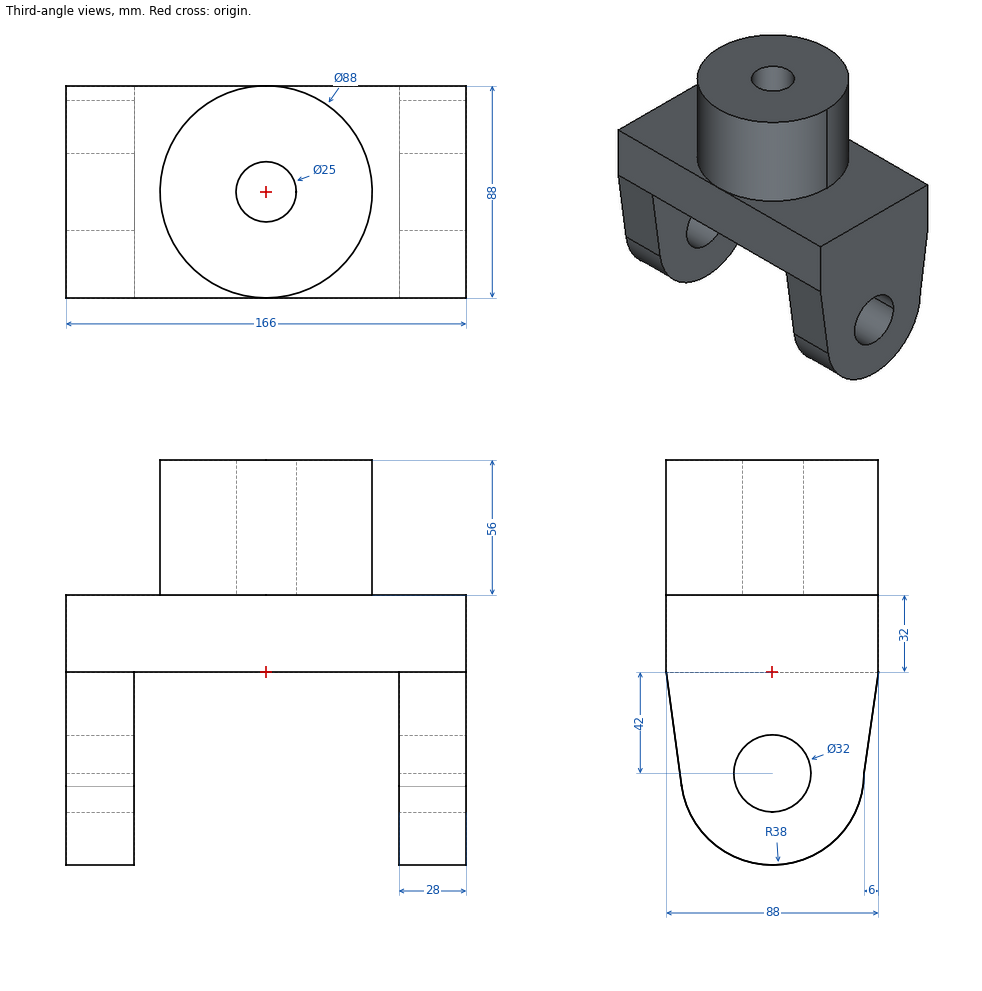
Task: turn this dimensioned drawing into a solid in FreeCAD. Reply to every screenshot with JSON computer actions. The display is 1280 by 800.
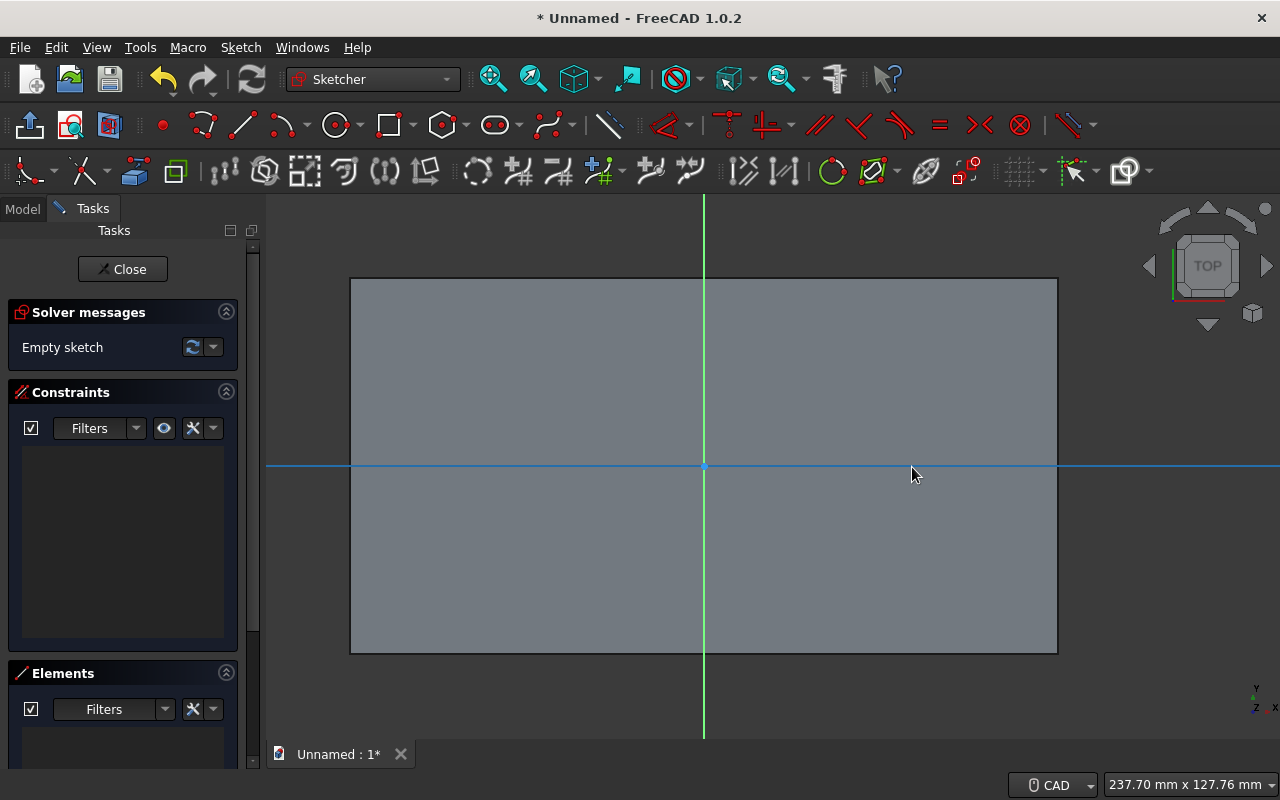
{"action": "left_click", "coordinate": [336, 126]}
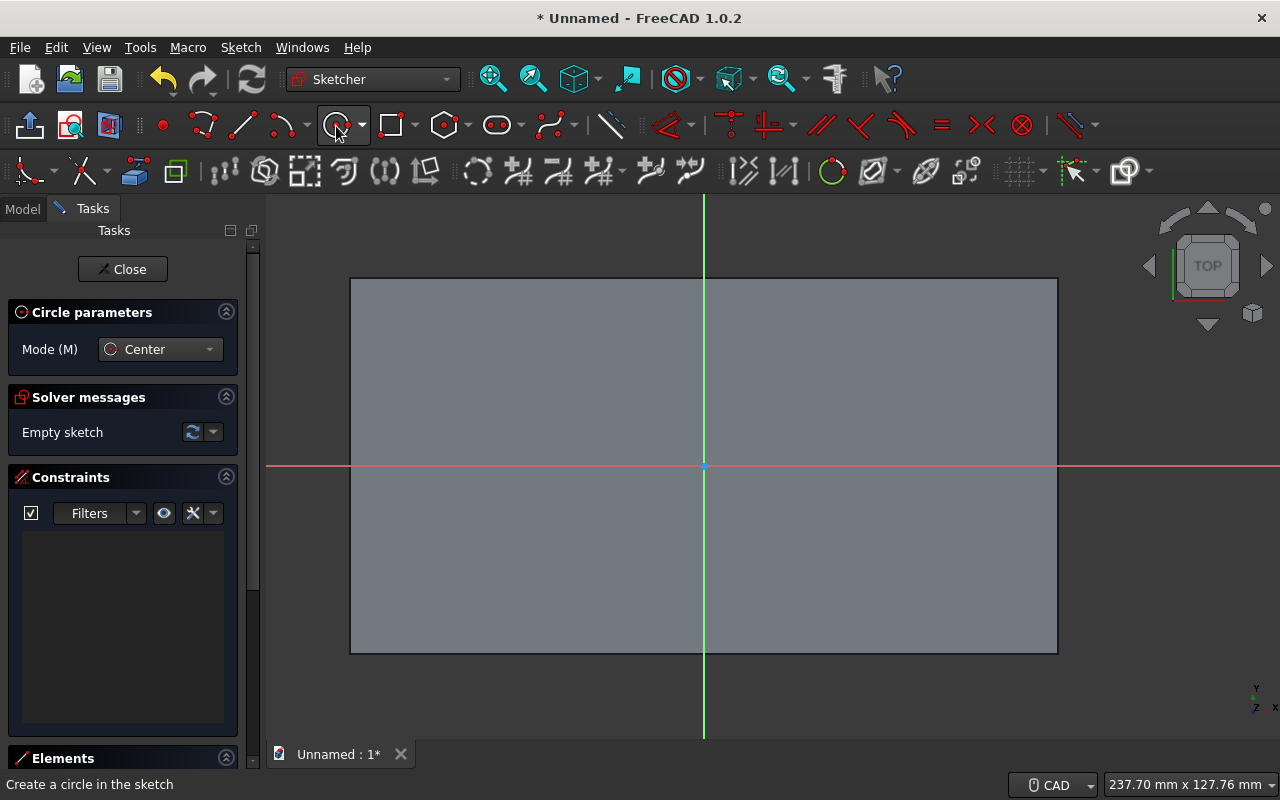
{"action": "left_click", "coordinate": [704, 466]}
{"action": "left_click", "coordinate": [837, 333]}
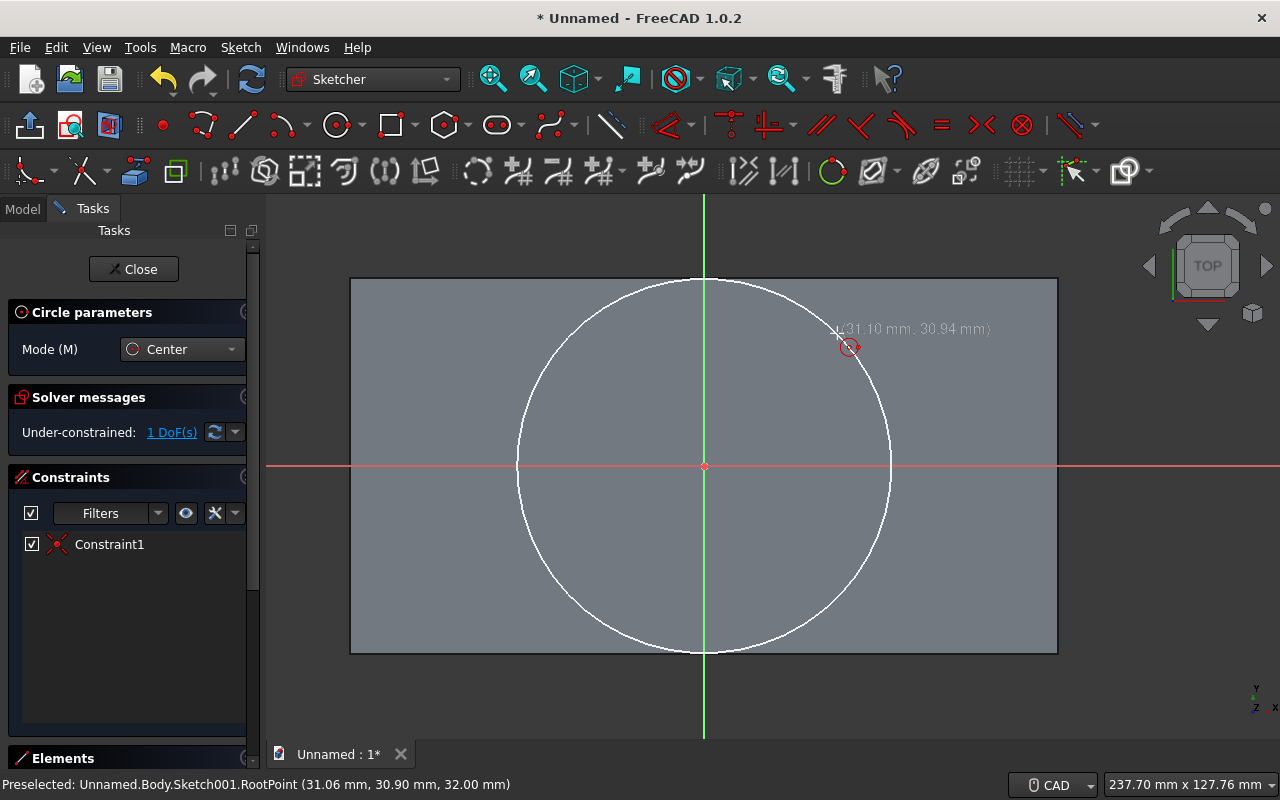
{"action": "left_click", "coordinate": [704, 466]}
{"action": "left_click", "coordinate": [742, 428]}
{"action": "key", "text": "Escape"}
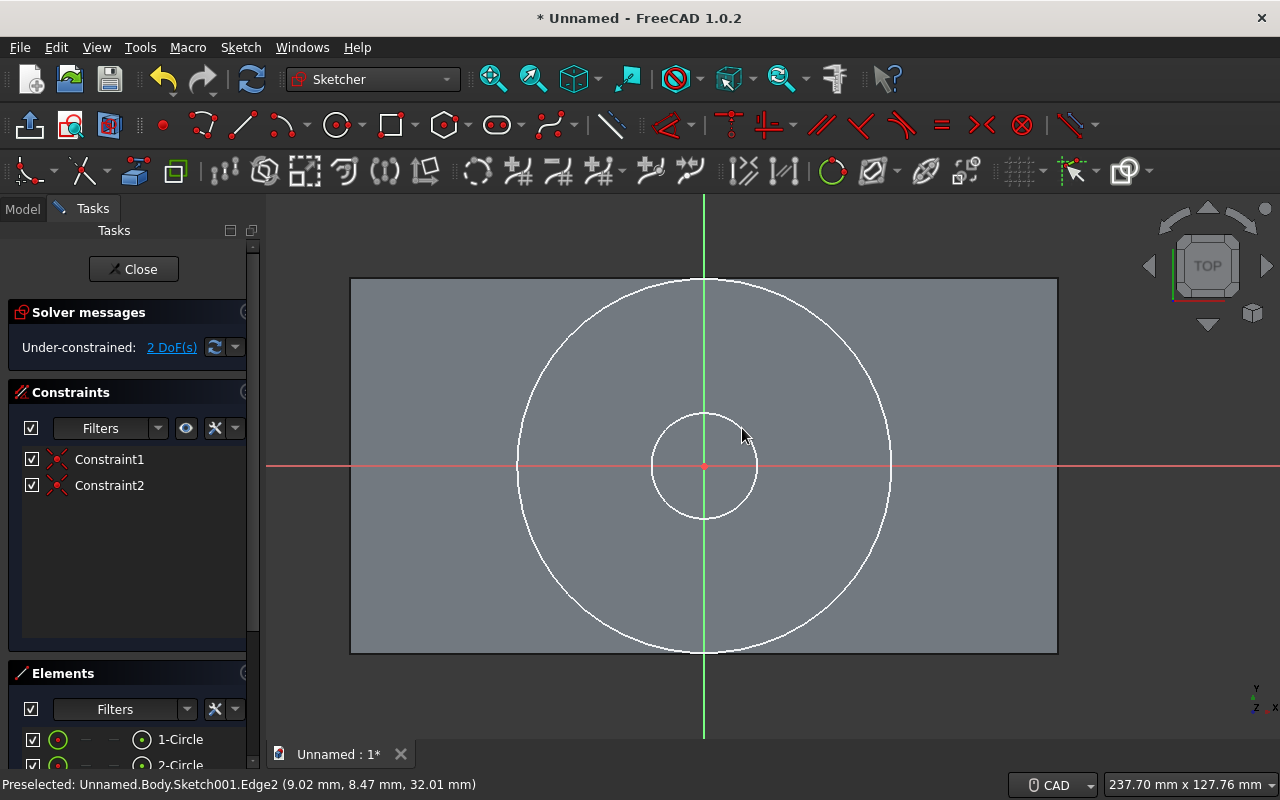
{"action": "left_click", "coordinate": [666, 126]}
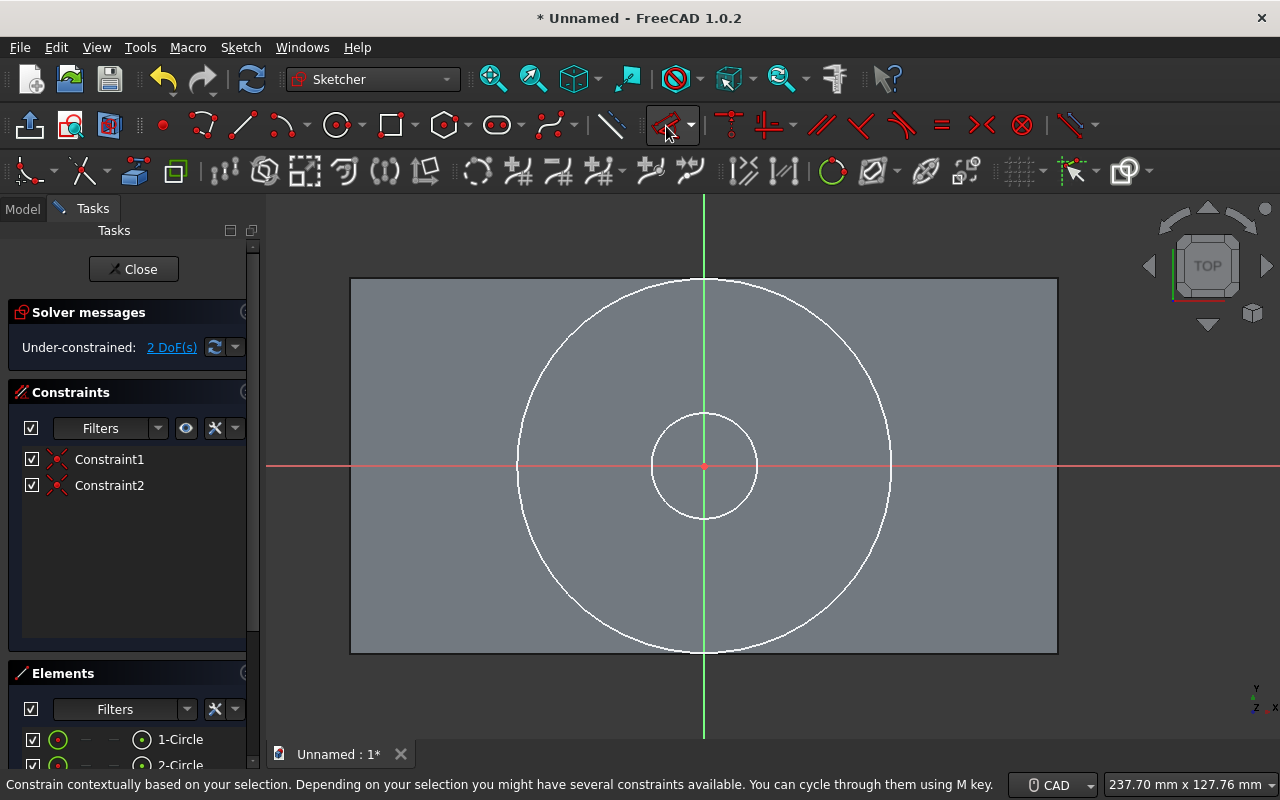
{"action": "left_click", "coordinate": [836, 333]}
{"action": "left_click", "coordinate": [859, 310]}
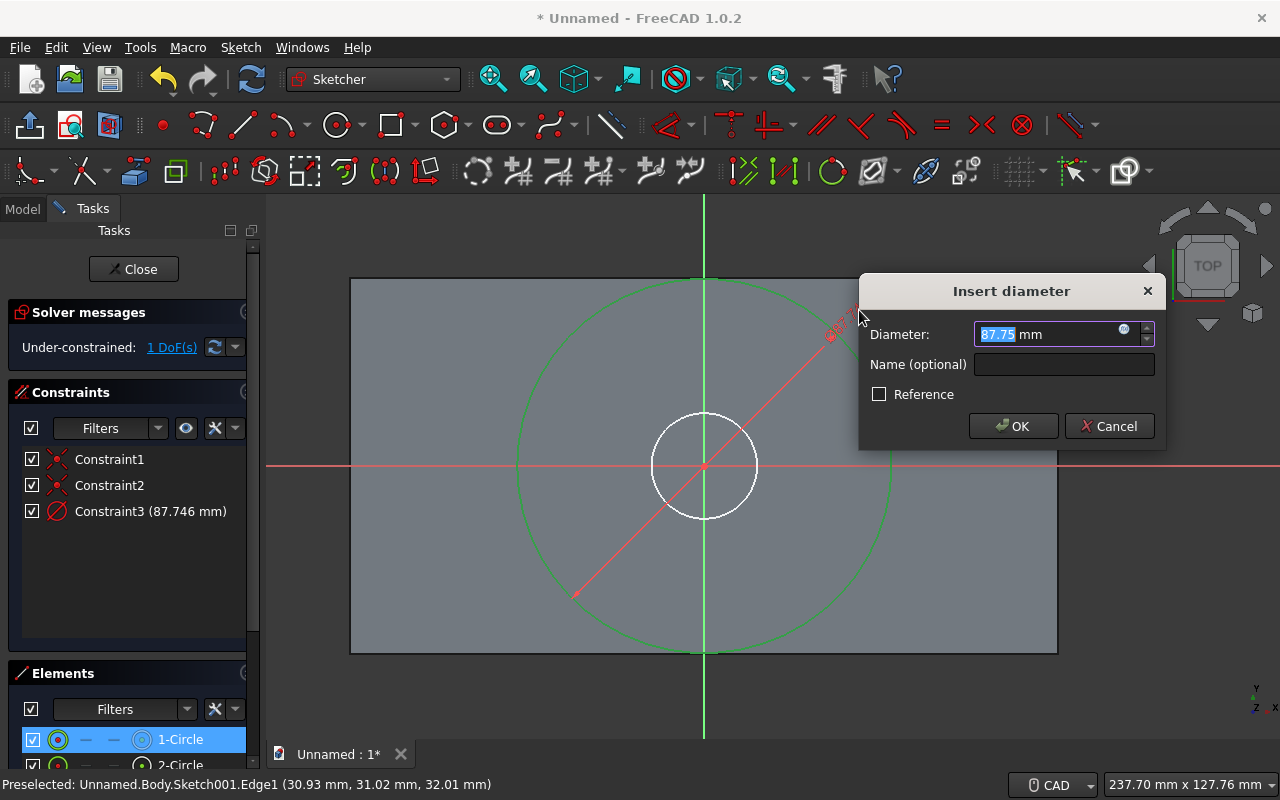
{"action": "type", "text": "88"}
{"action": "key", "text": "Return"}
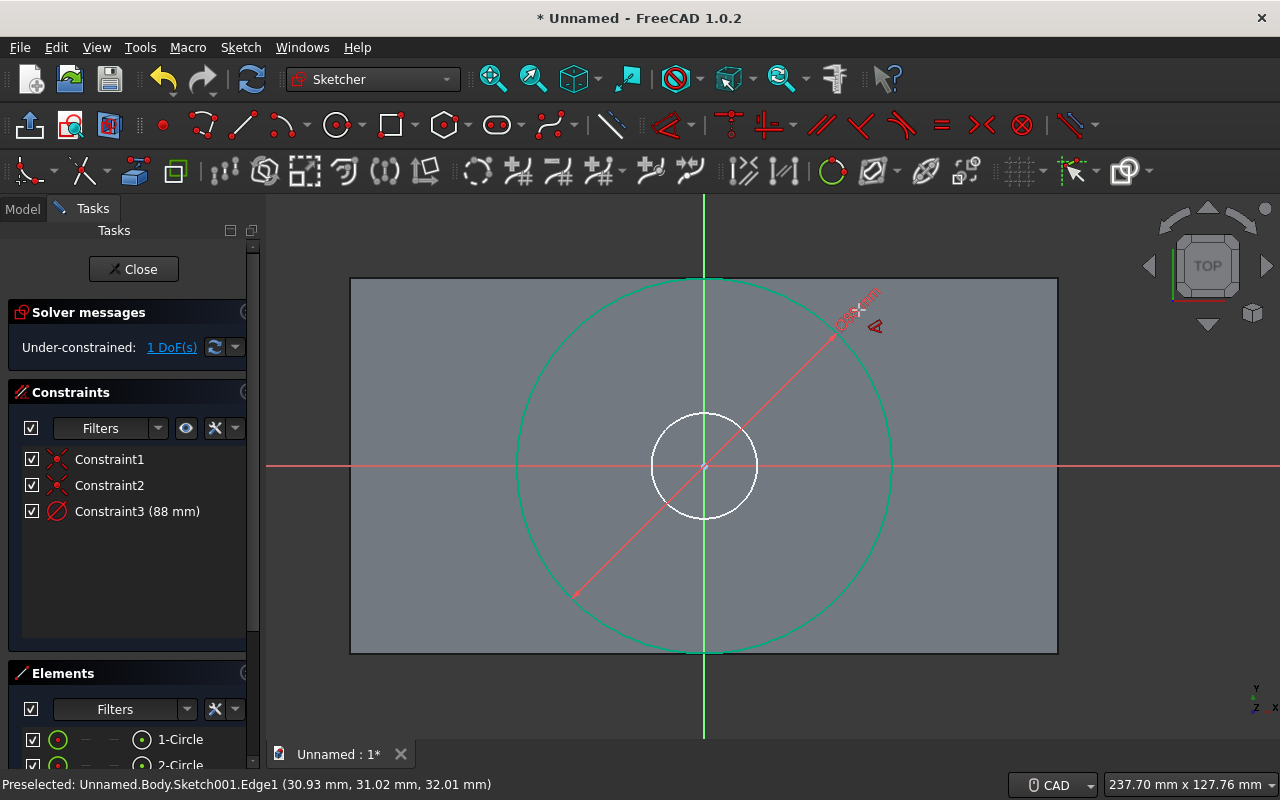
{"action": "left_click", "coordinate": [742, 429]}
{"action": "left_click", "coordinate": [765, 407]}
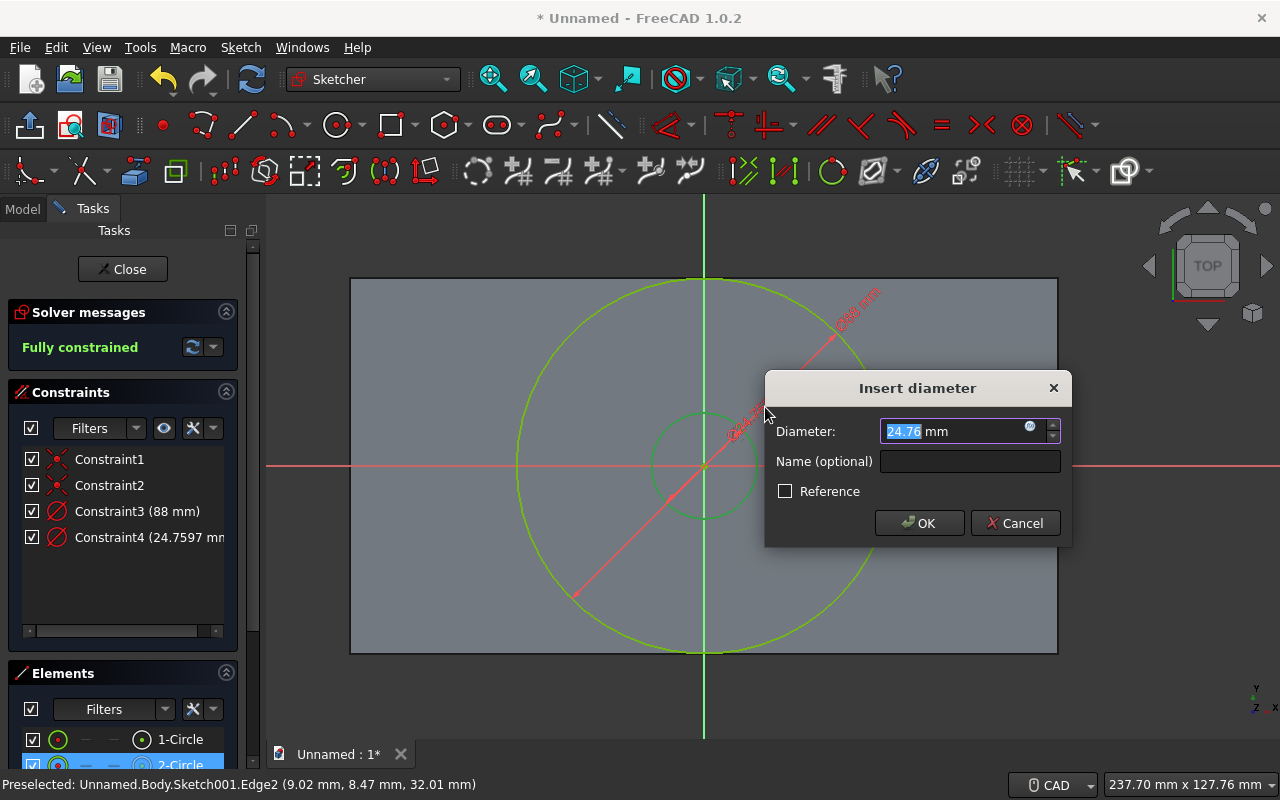
{"action": "type", "text": "25"}
{"action": "key", "text": "Return"}
{"action": "key", "text": "Escape"}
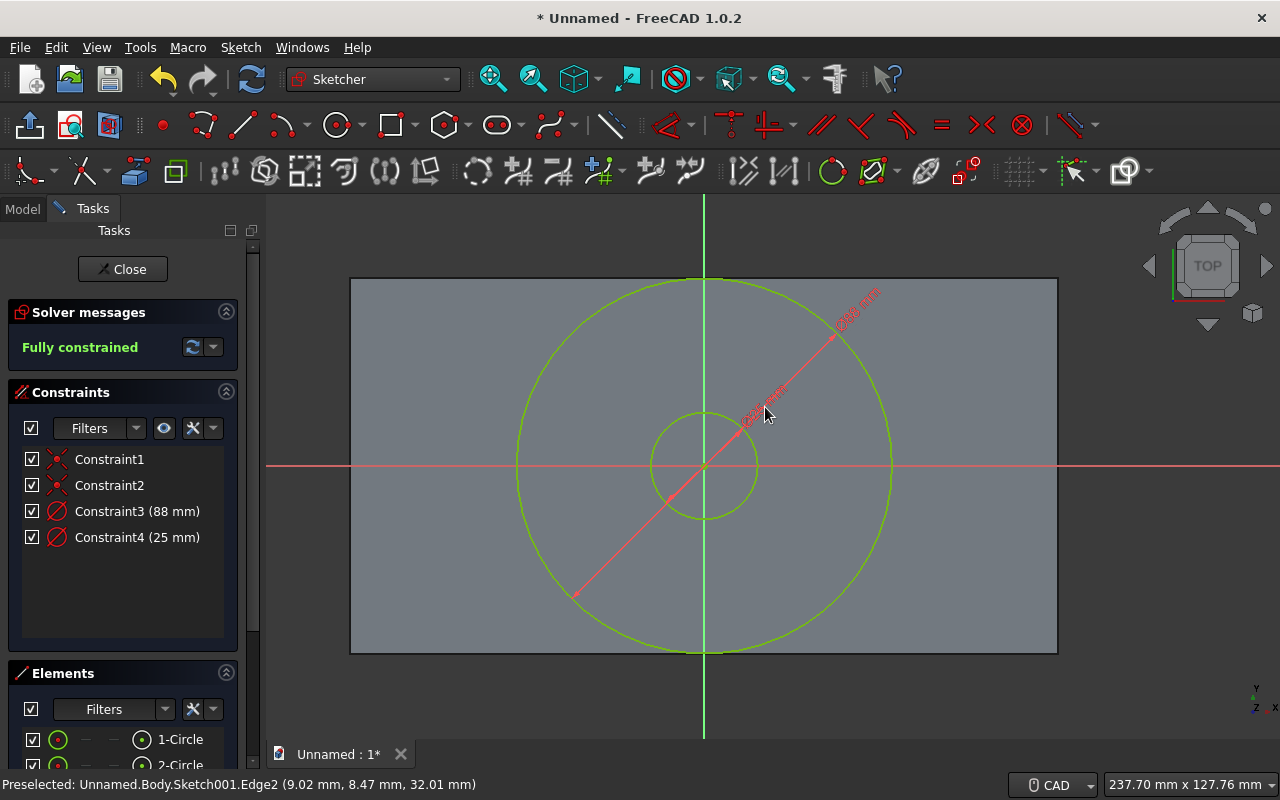
{"action": "left_click", "coordinate": [123, 269]}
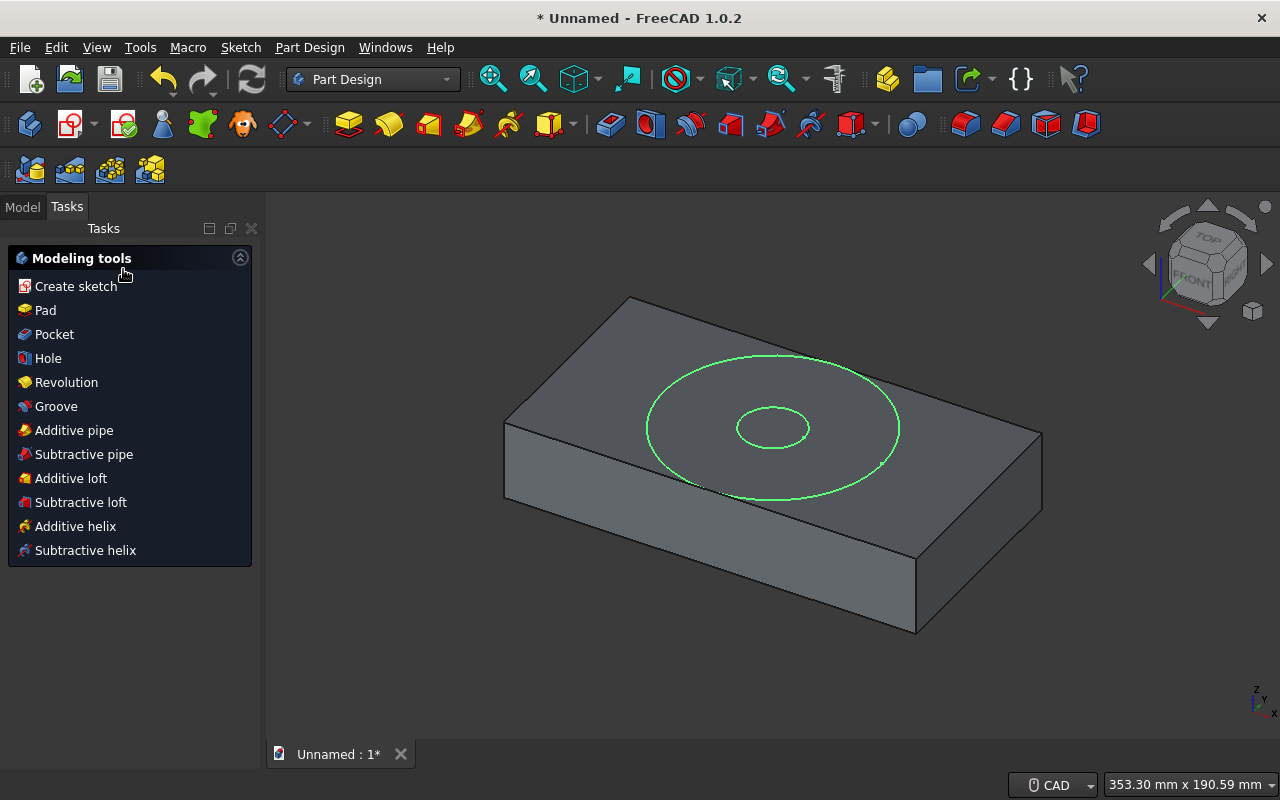
{"action": "left_click", "coordinate": [350, 124]}